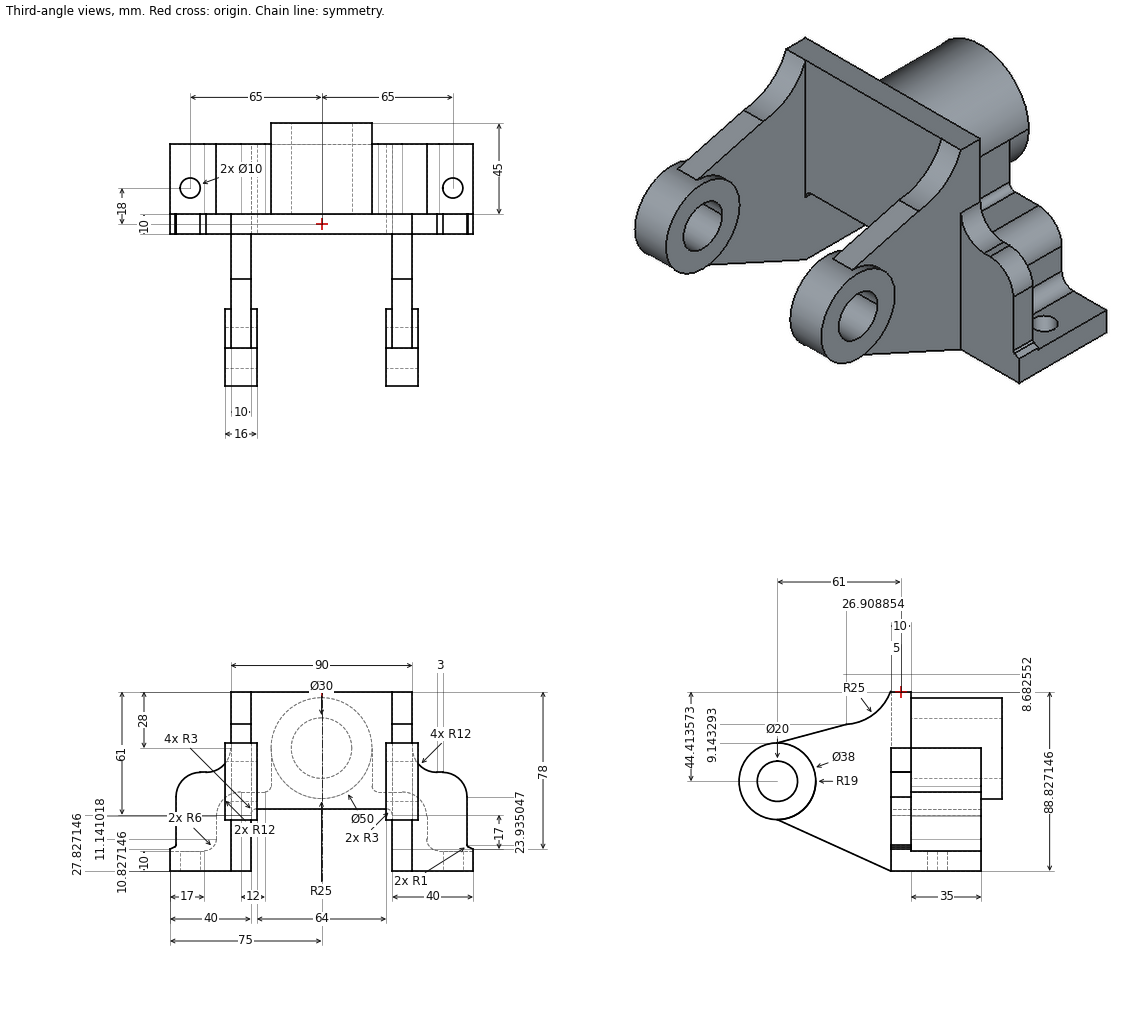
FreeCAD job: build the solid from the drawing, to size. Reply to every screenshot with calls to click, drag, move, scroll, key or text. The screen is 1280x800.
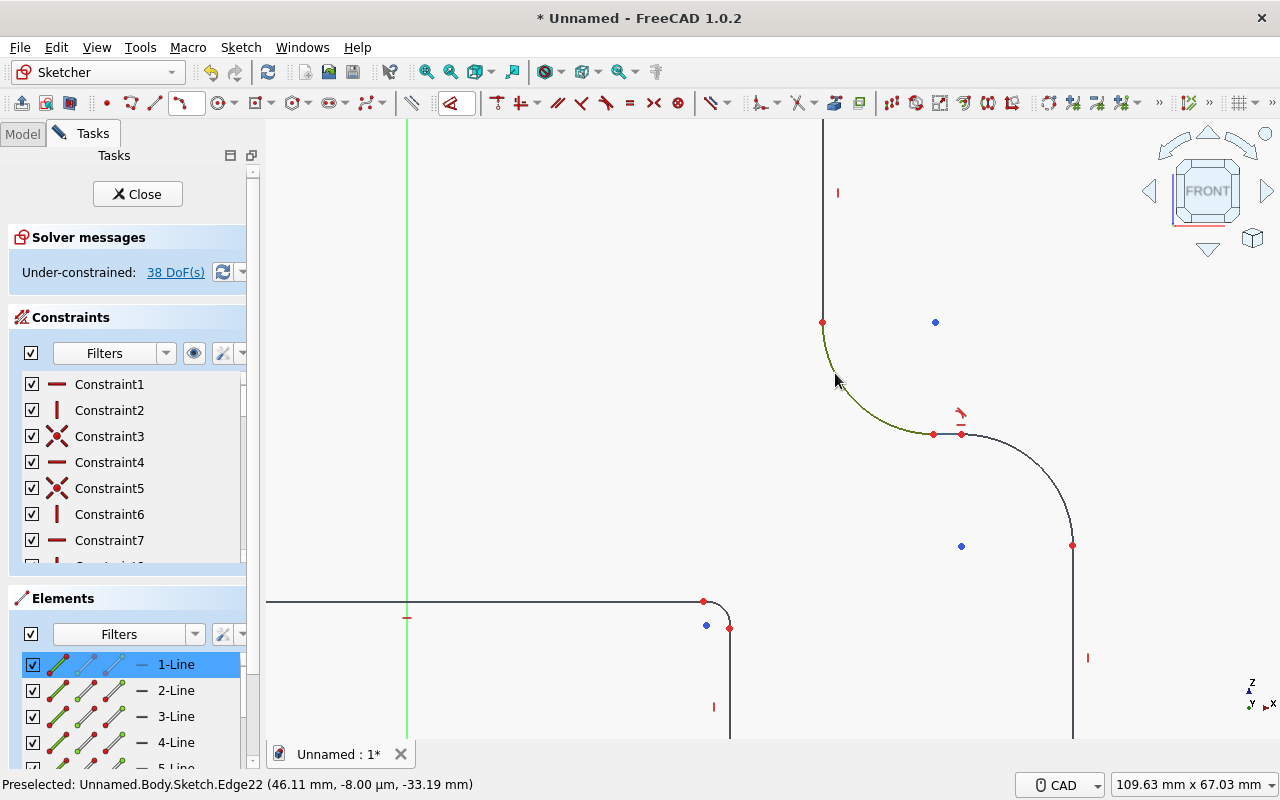
key(t)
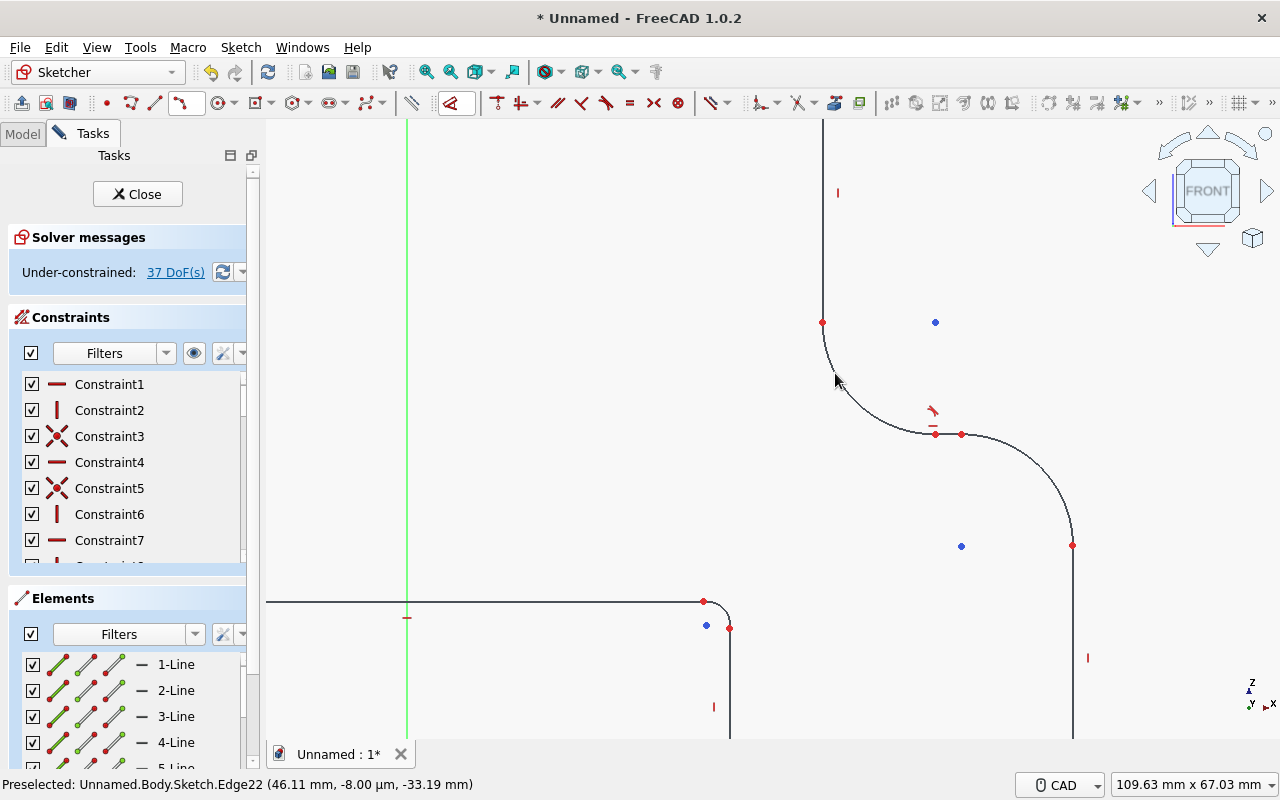
click(1073, 613)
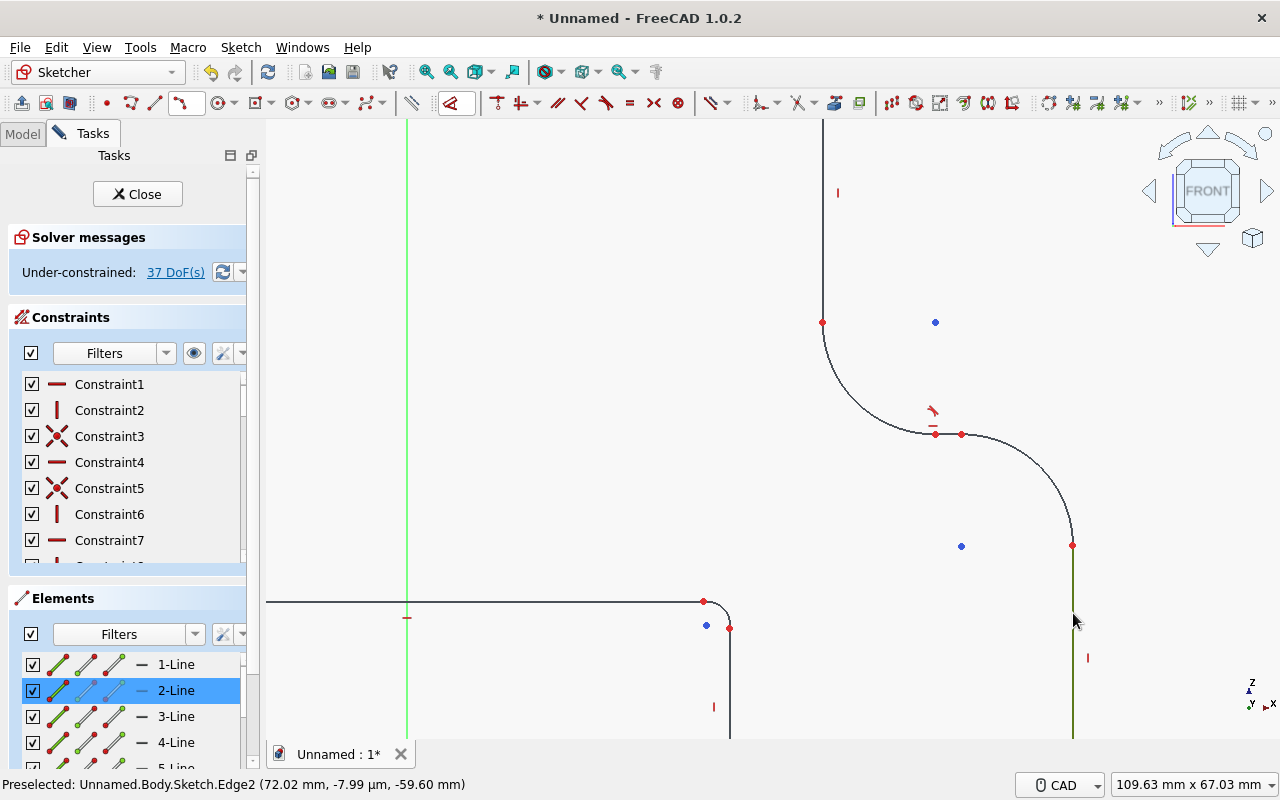
click(1061, 495)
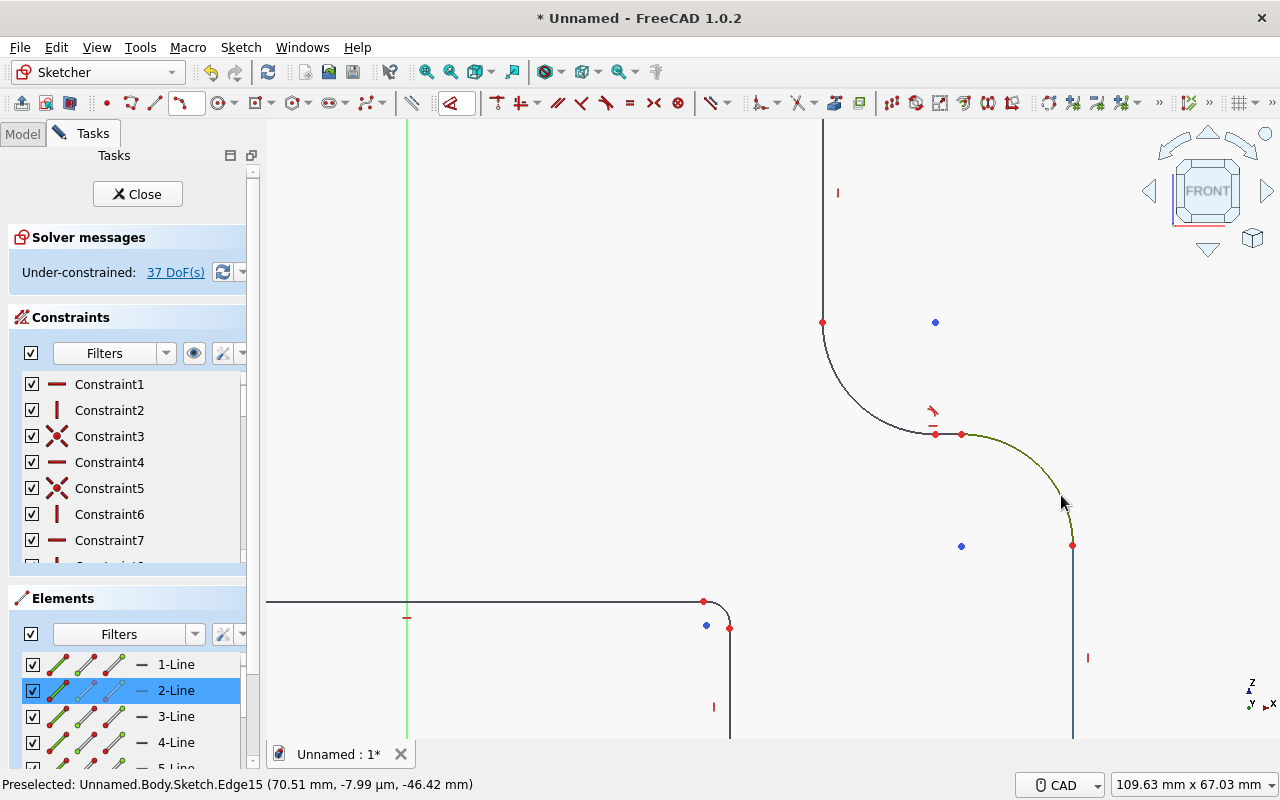
key(t)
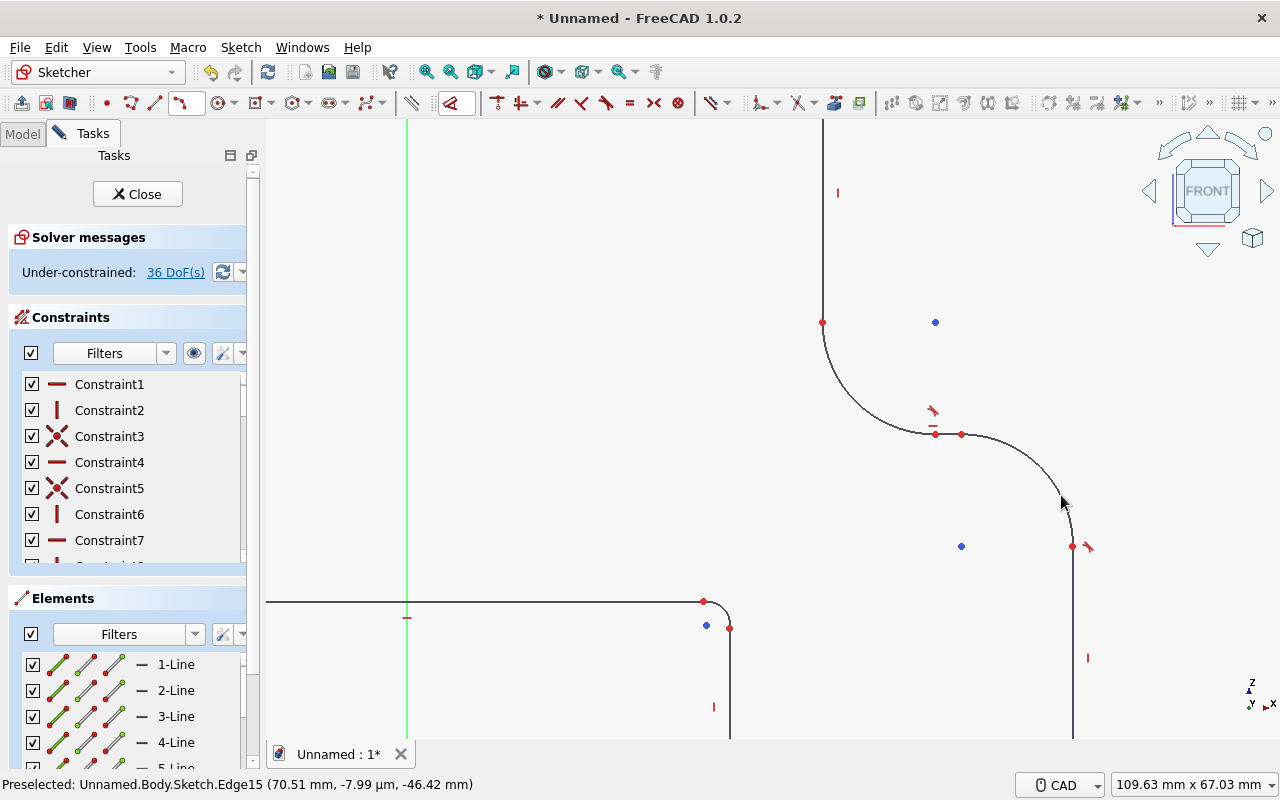
click(1073, 613)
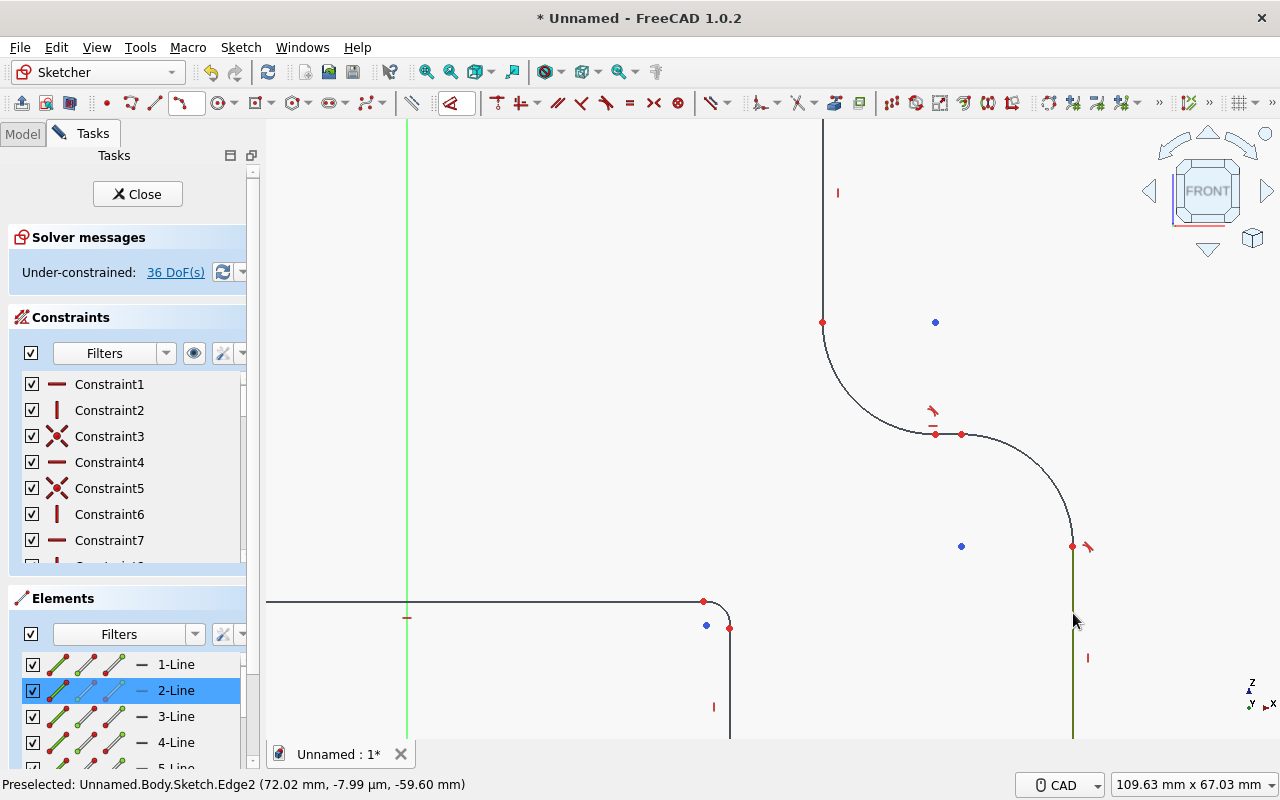
scroll(947, 434, down, 4)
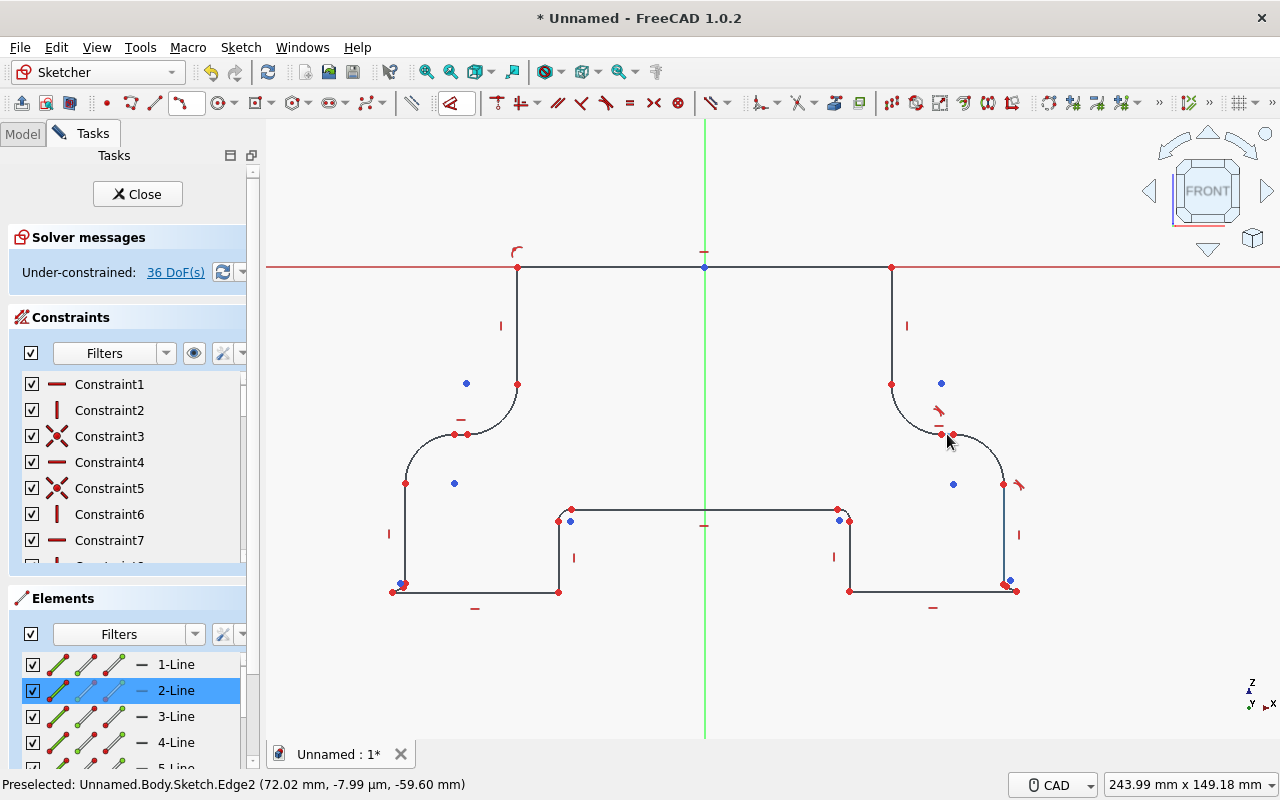
scroll(1005, 586, up, 11)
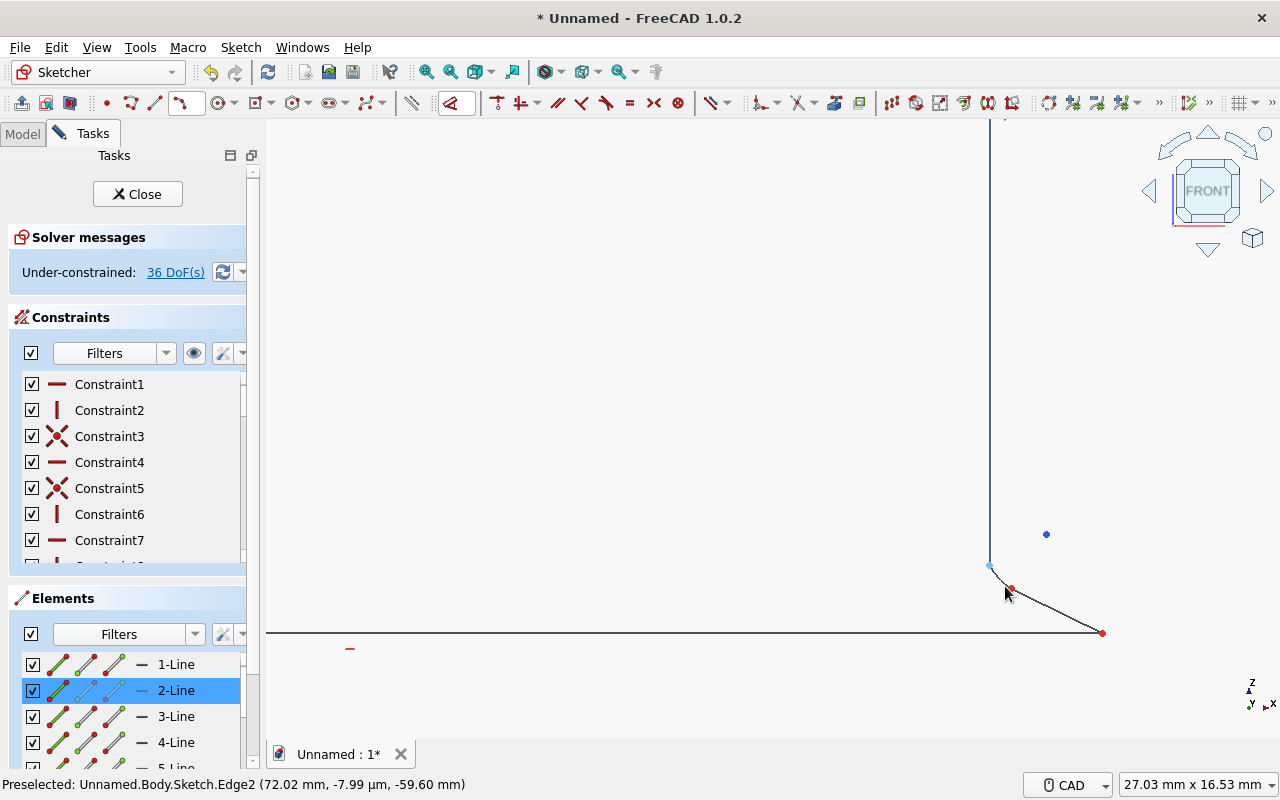
click(999, 579)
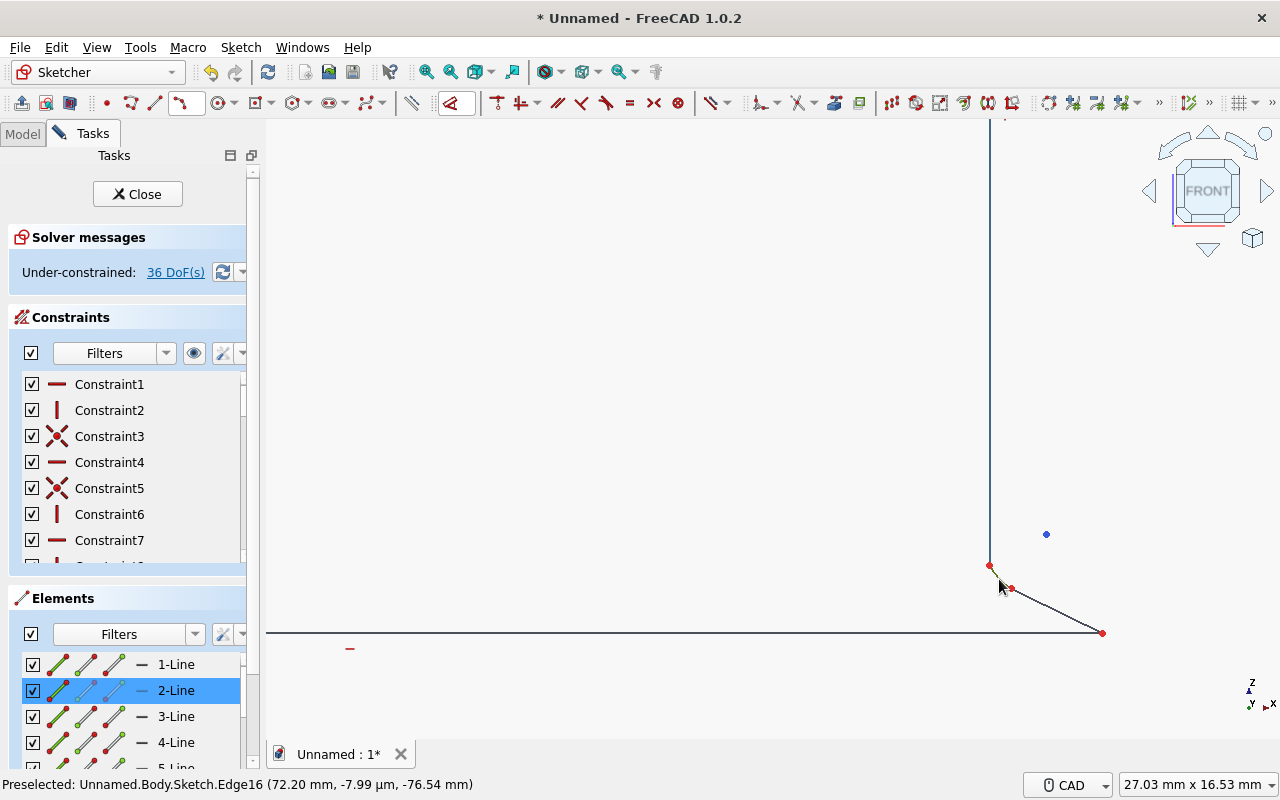
key(t)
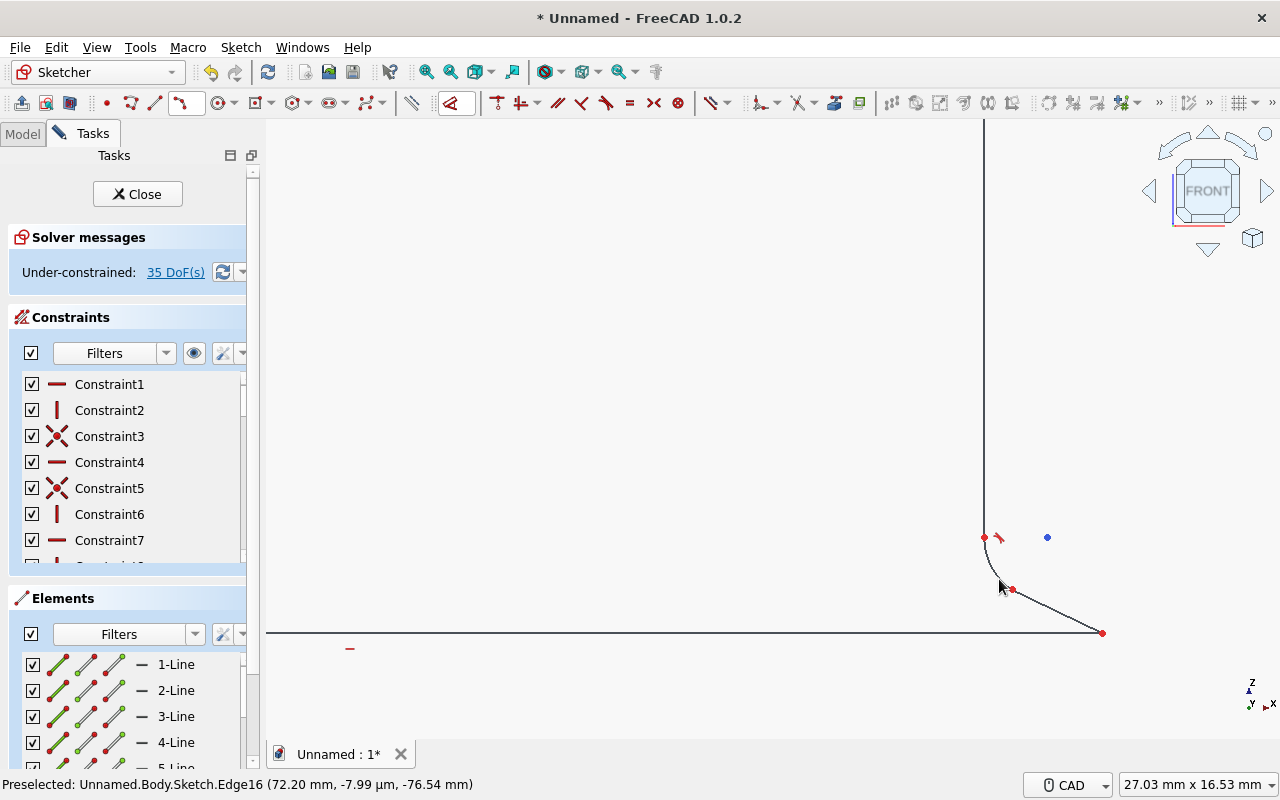
click(1039, 603)